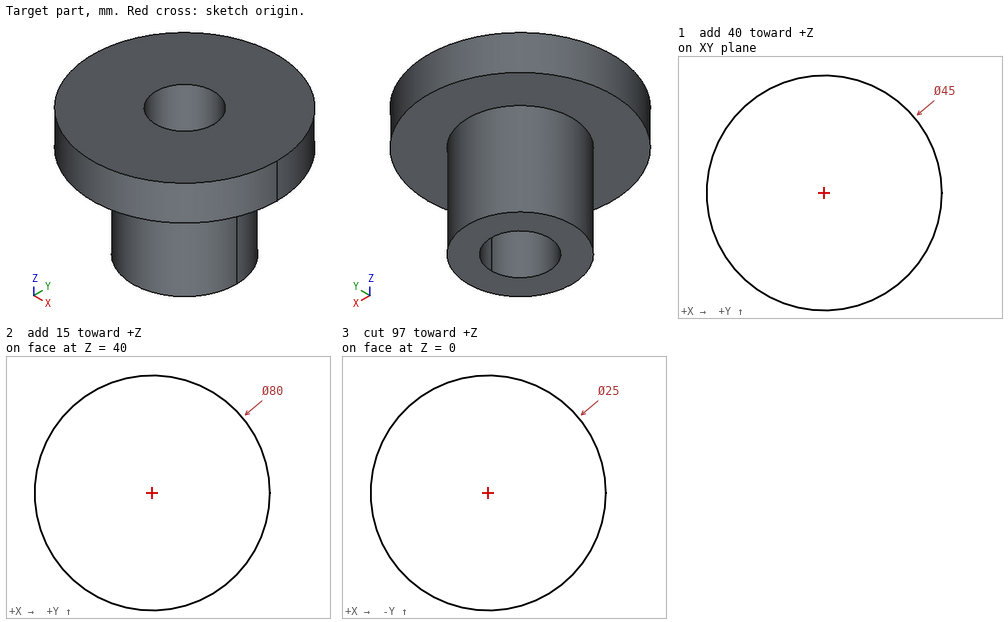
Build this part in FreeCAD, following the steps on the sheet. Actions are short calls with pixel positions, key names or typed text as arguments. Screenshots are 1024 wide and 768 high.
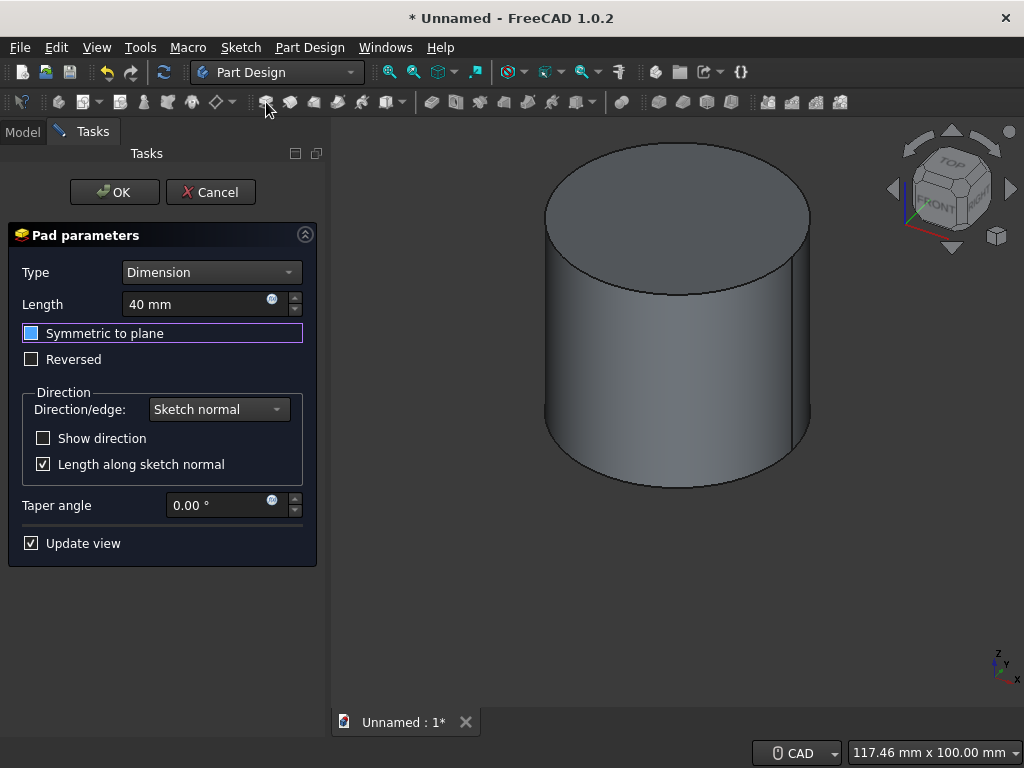
click(115, 192)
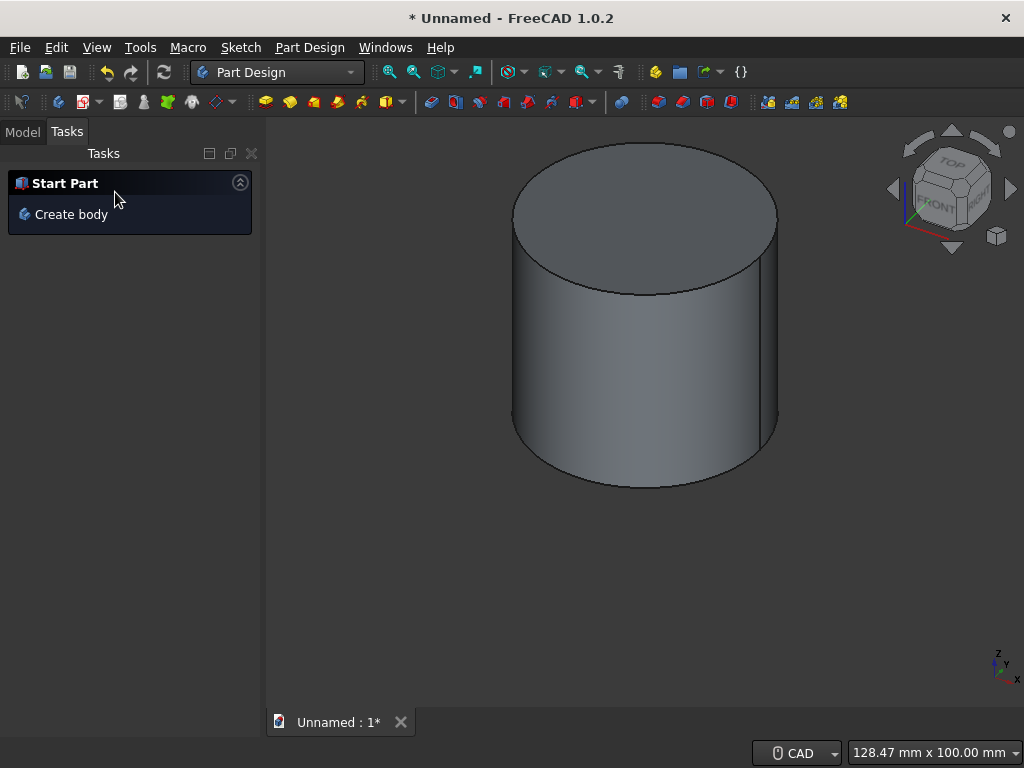
click(390, 72)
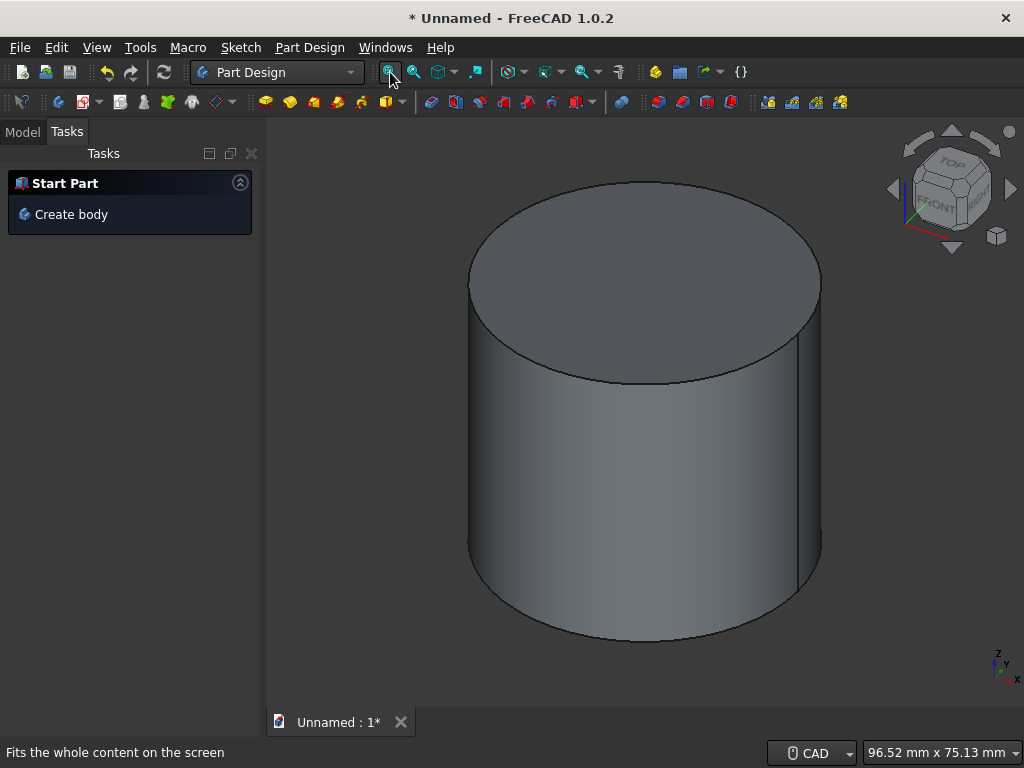
click(645, 282)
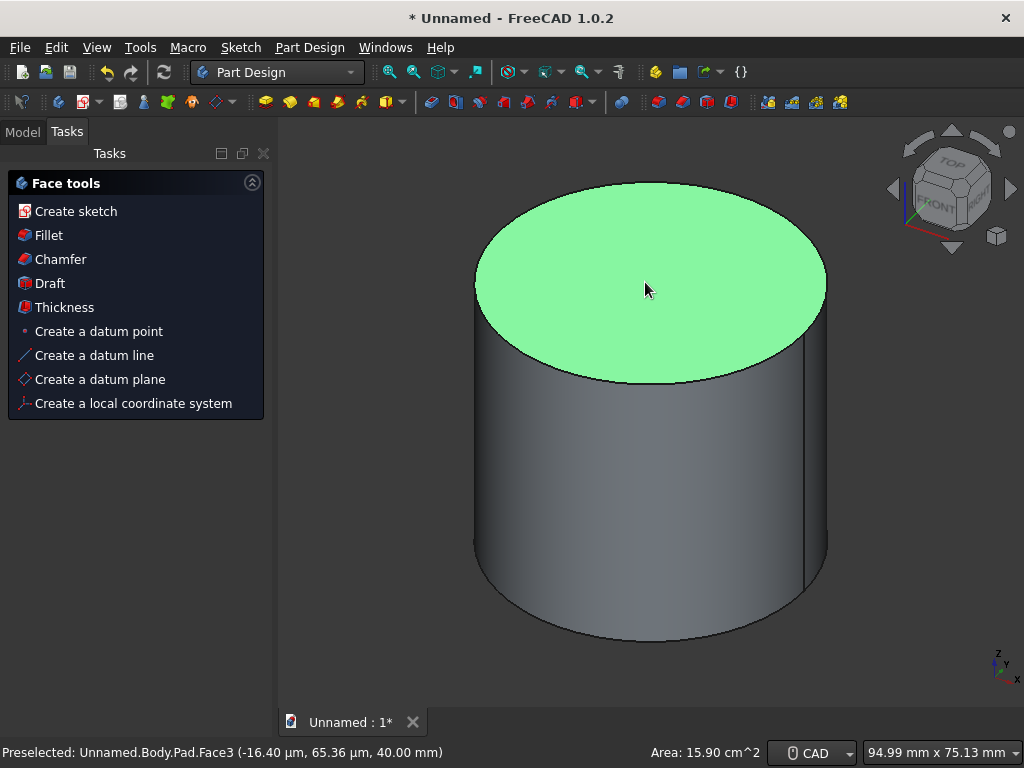
click(84, 102)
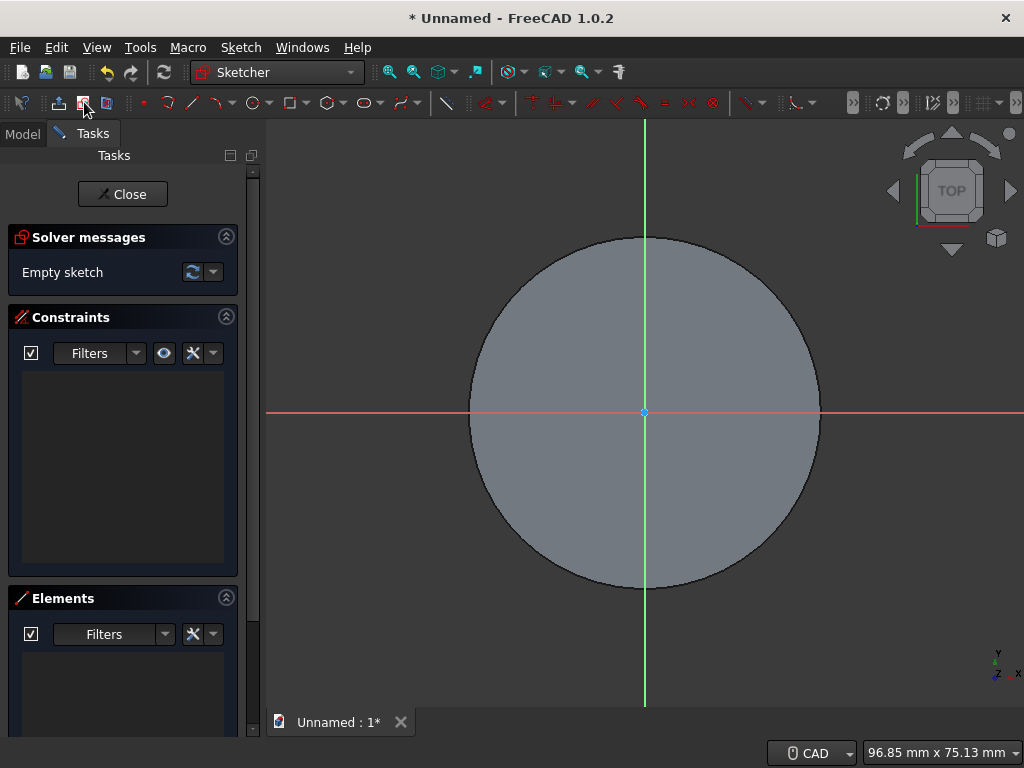
scroll(493, 413, down, 3)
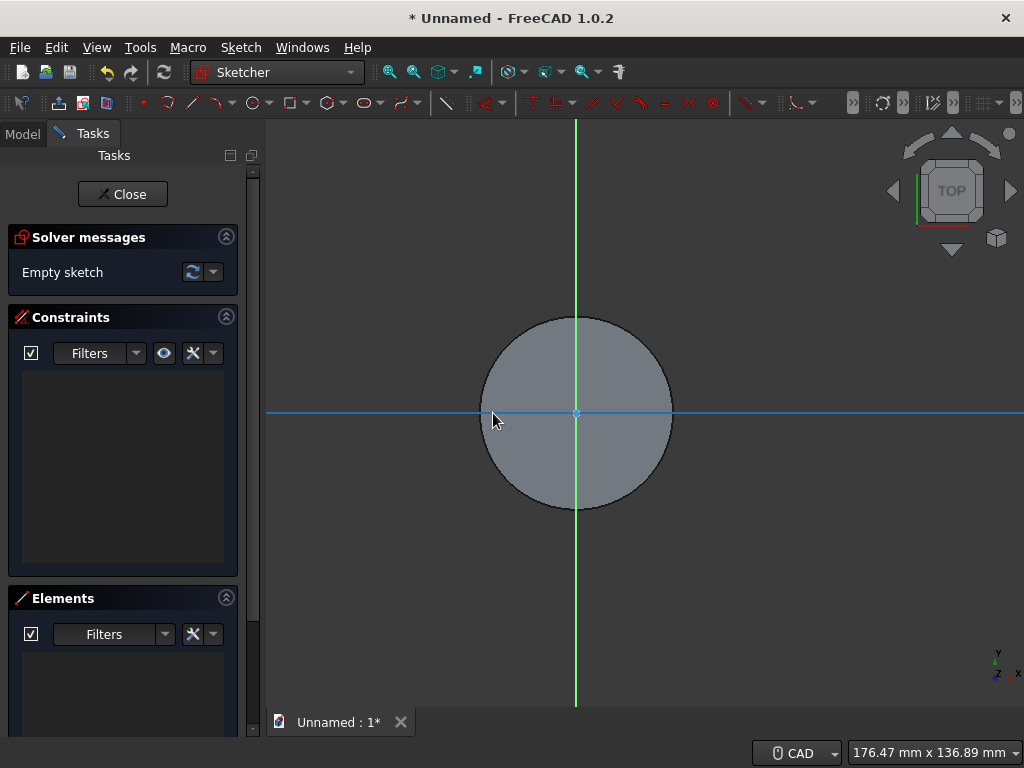
click(254, 104)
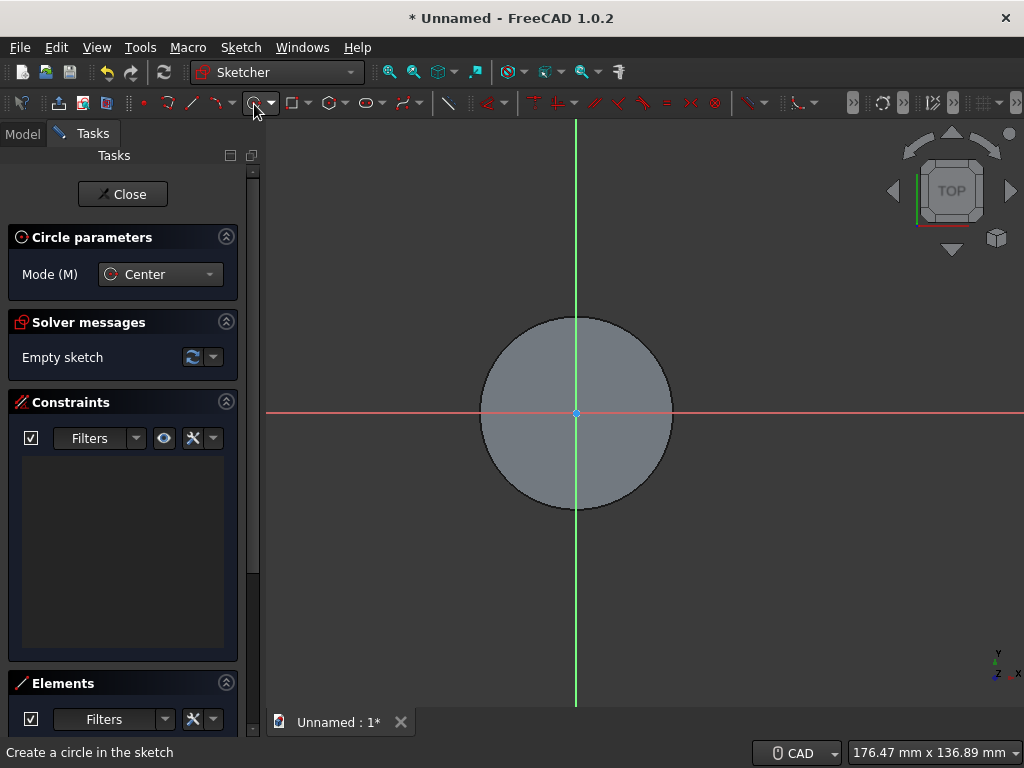
click(576, 413)
click(698, 292)
key(Escape)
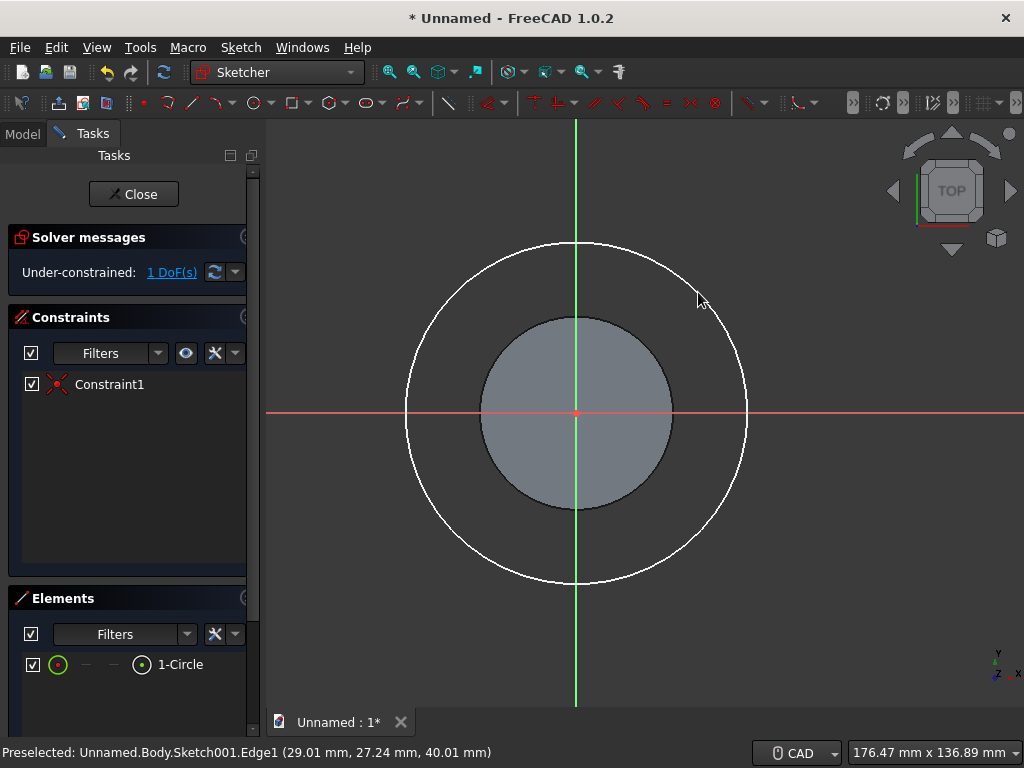
click(488, 104)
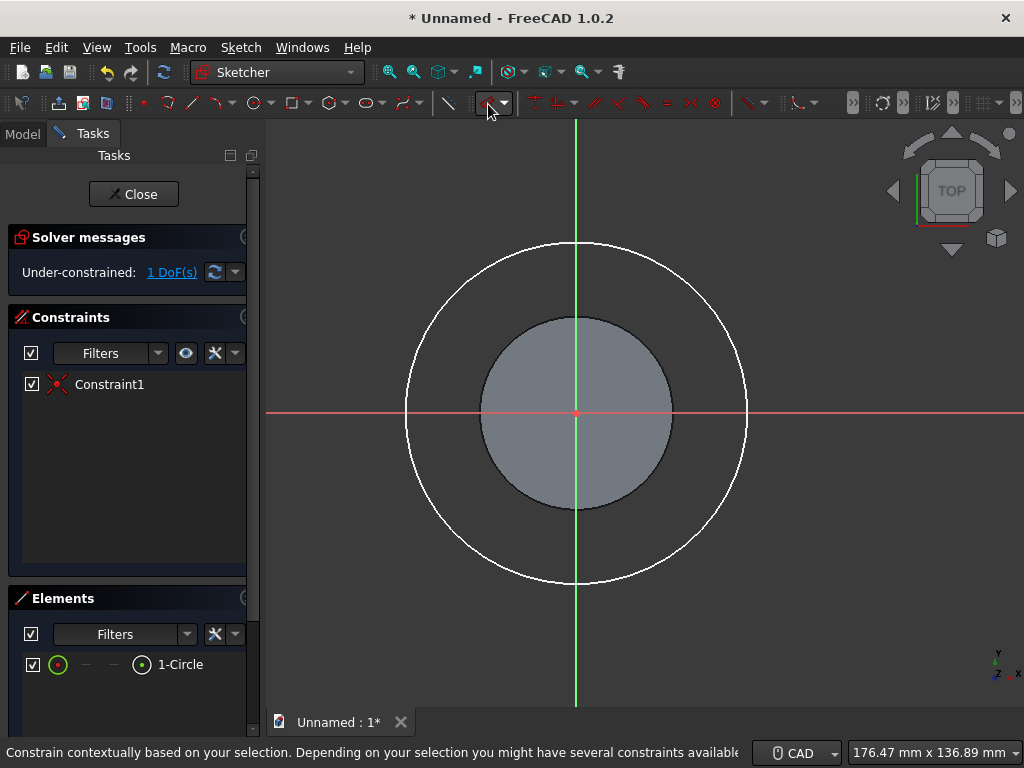
click(697, 292)
click(720, 269)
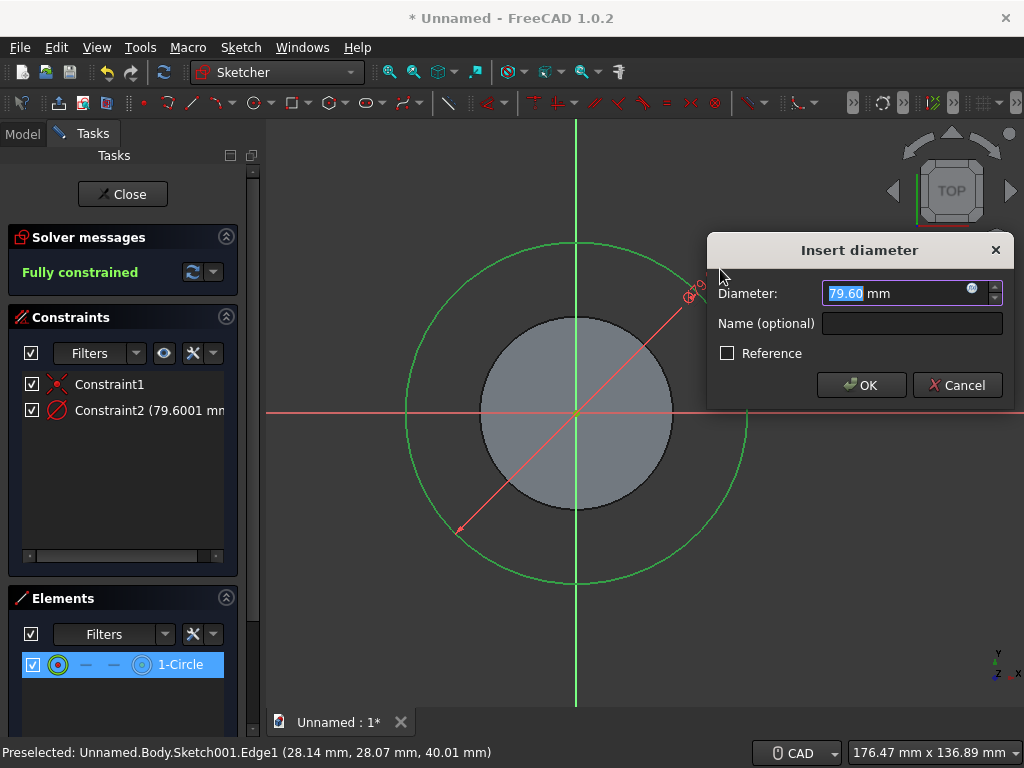
text(80)
key(Return)
key(Escape)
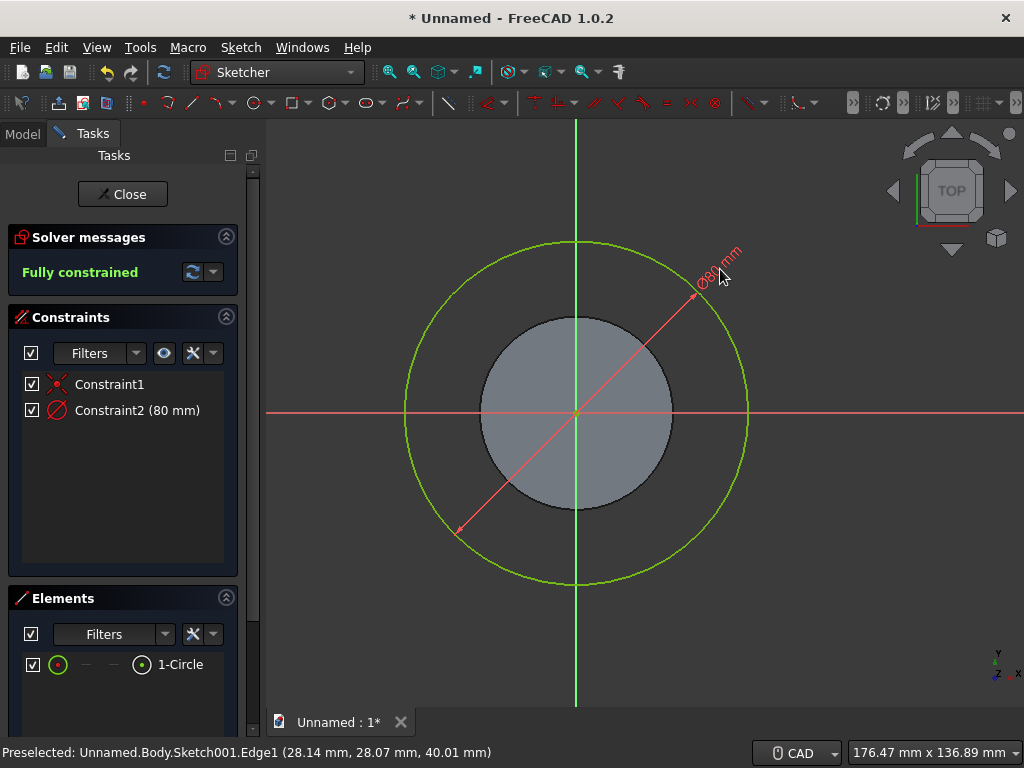
click(123, 194)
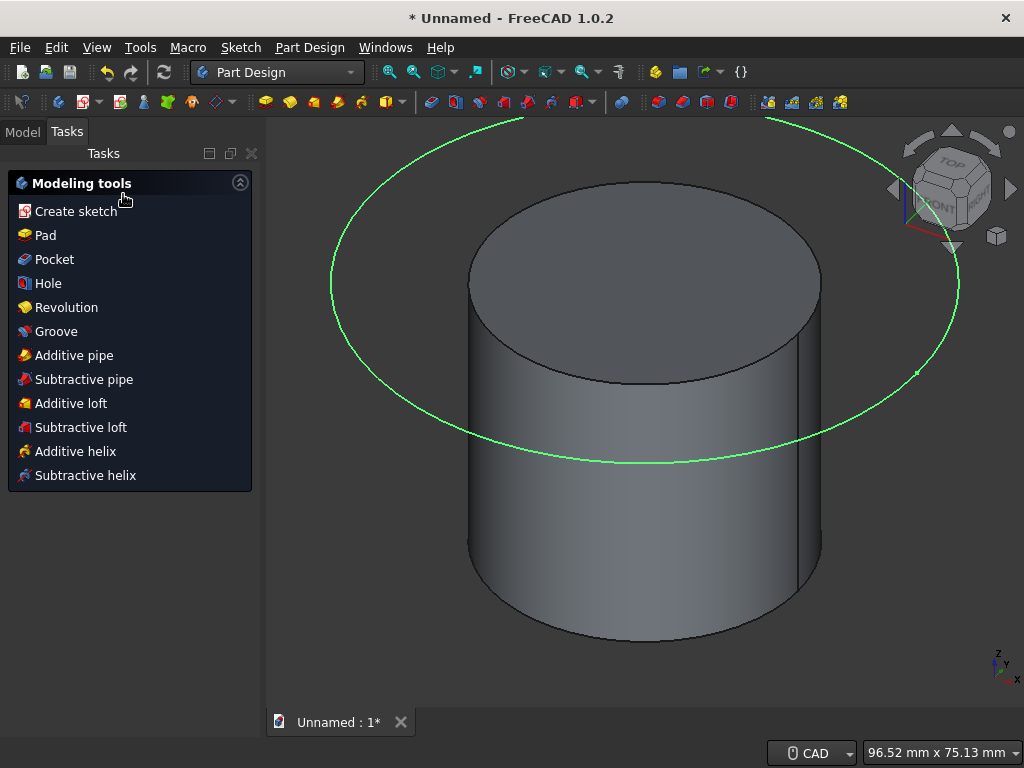
click(266, 102)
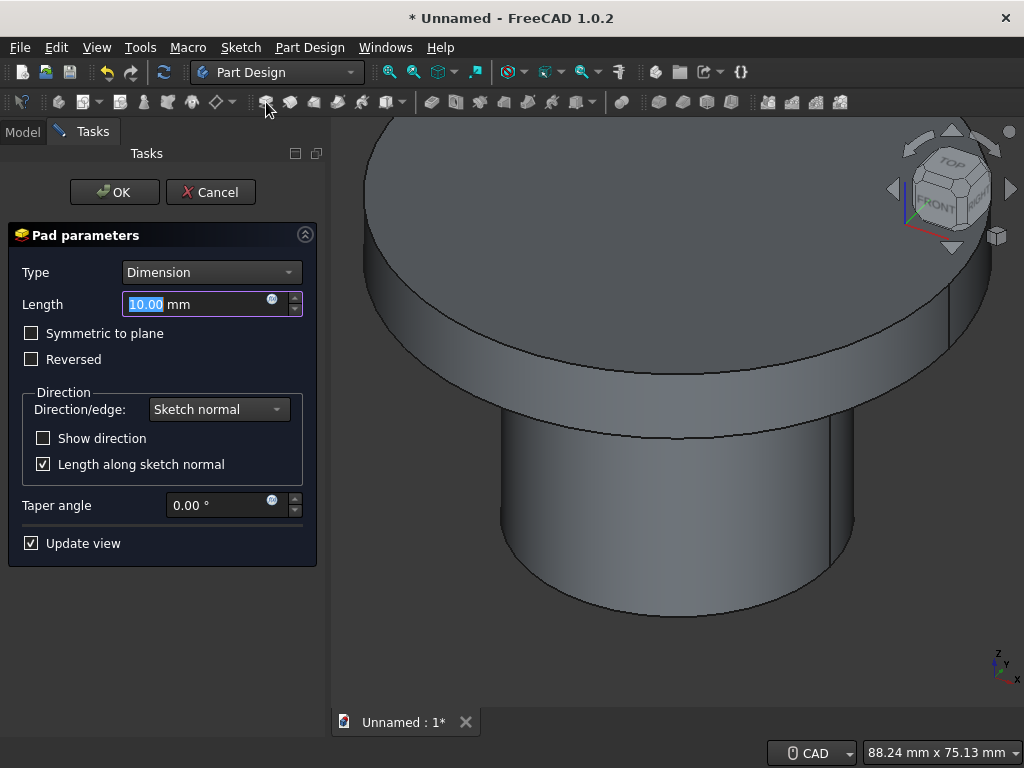
text(15)
key(Tab)